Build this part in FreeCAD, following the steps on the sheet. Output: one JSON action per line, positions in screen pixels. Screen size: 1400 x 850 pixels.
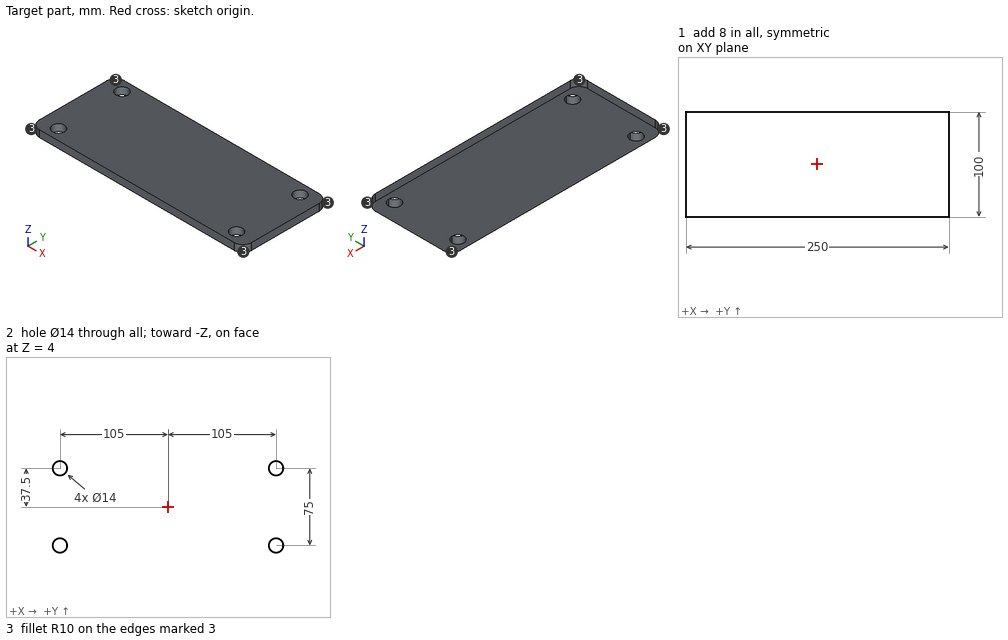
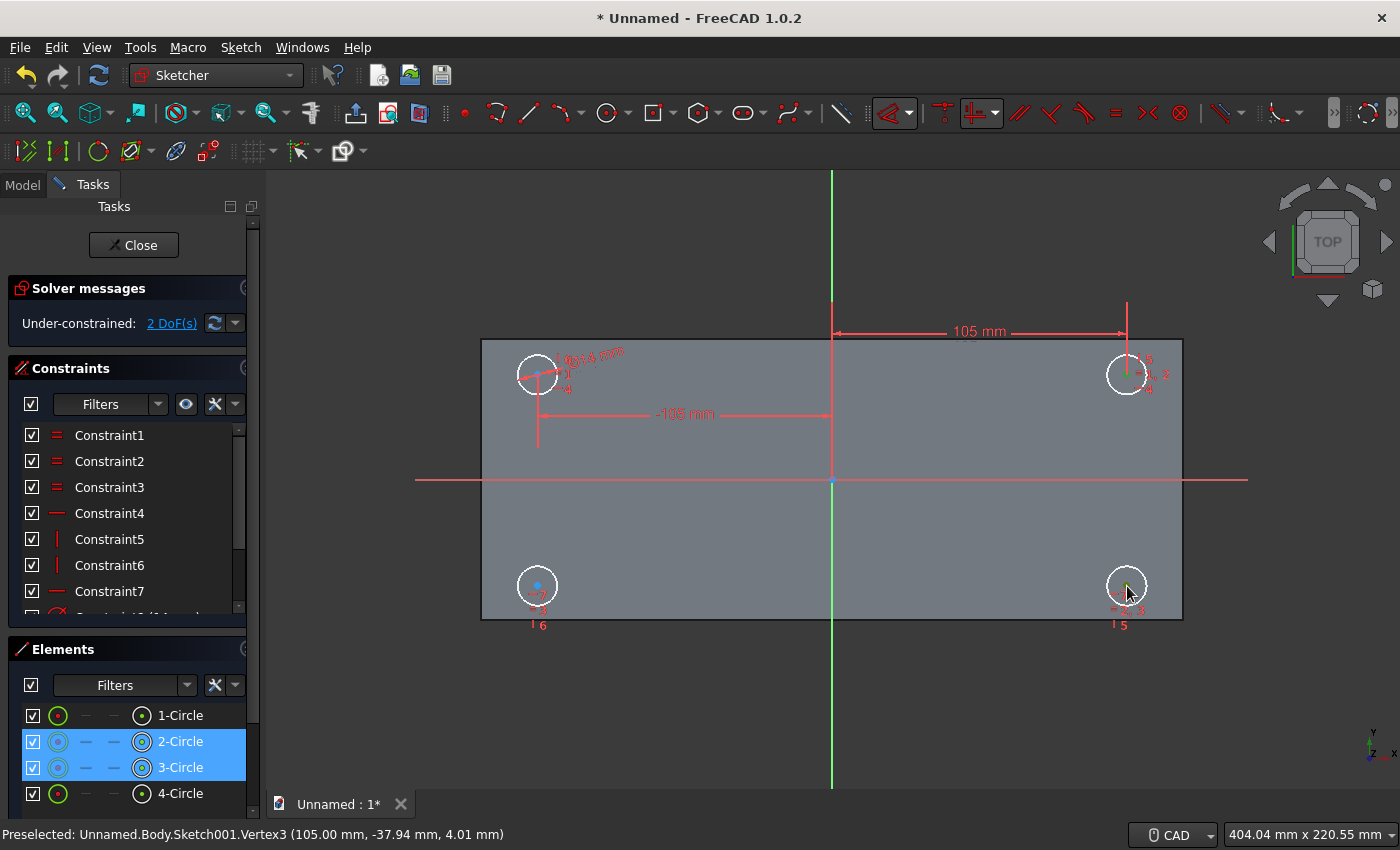
{"action": "left_click", "coordinate": [912, 114]}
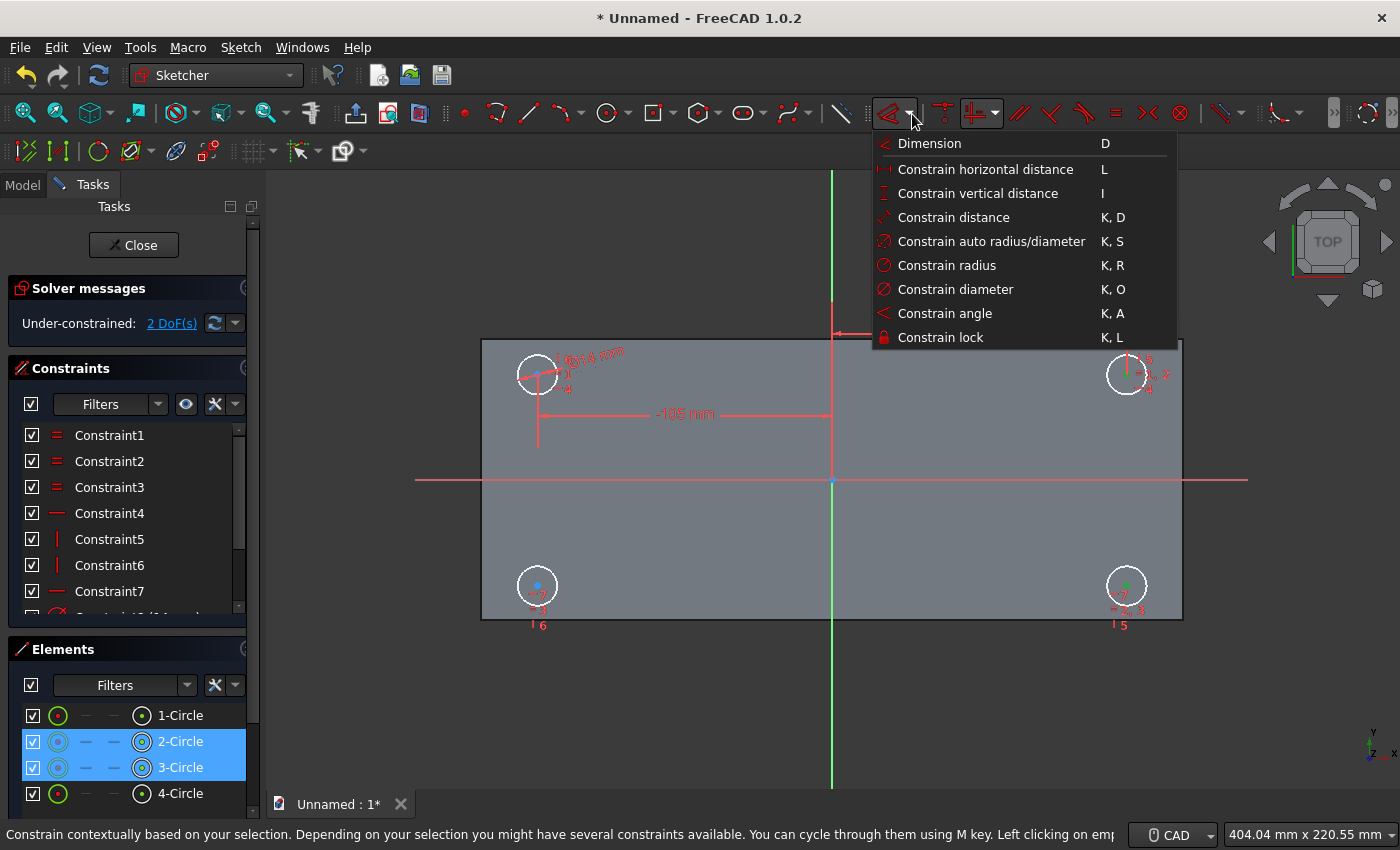
{"action": "left_click", "coordinate": [1025, 193]}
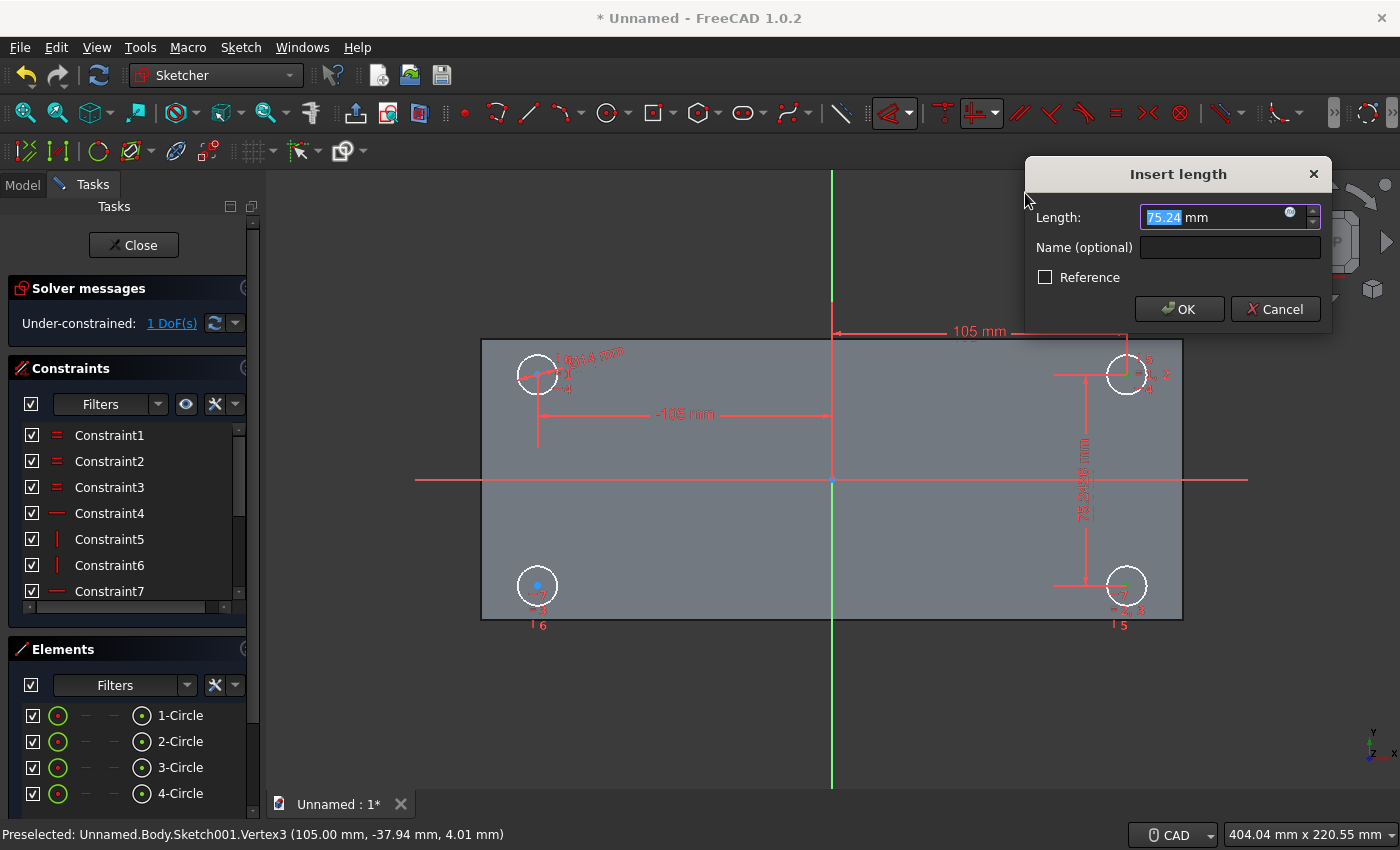
{"action": "type", "text": "75"}
{"action": "key", "text": "Return"}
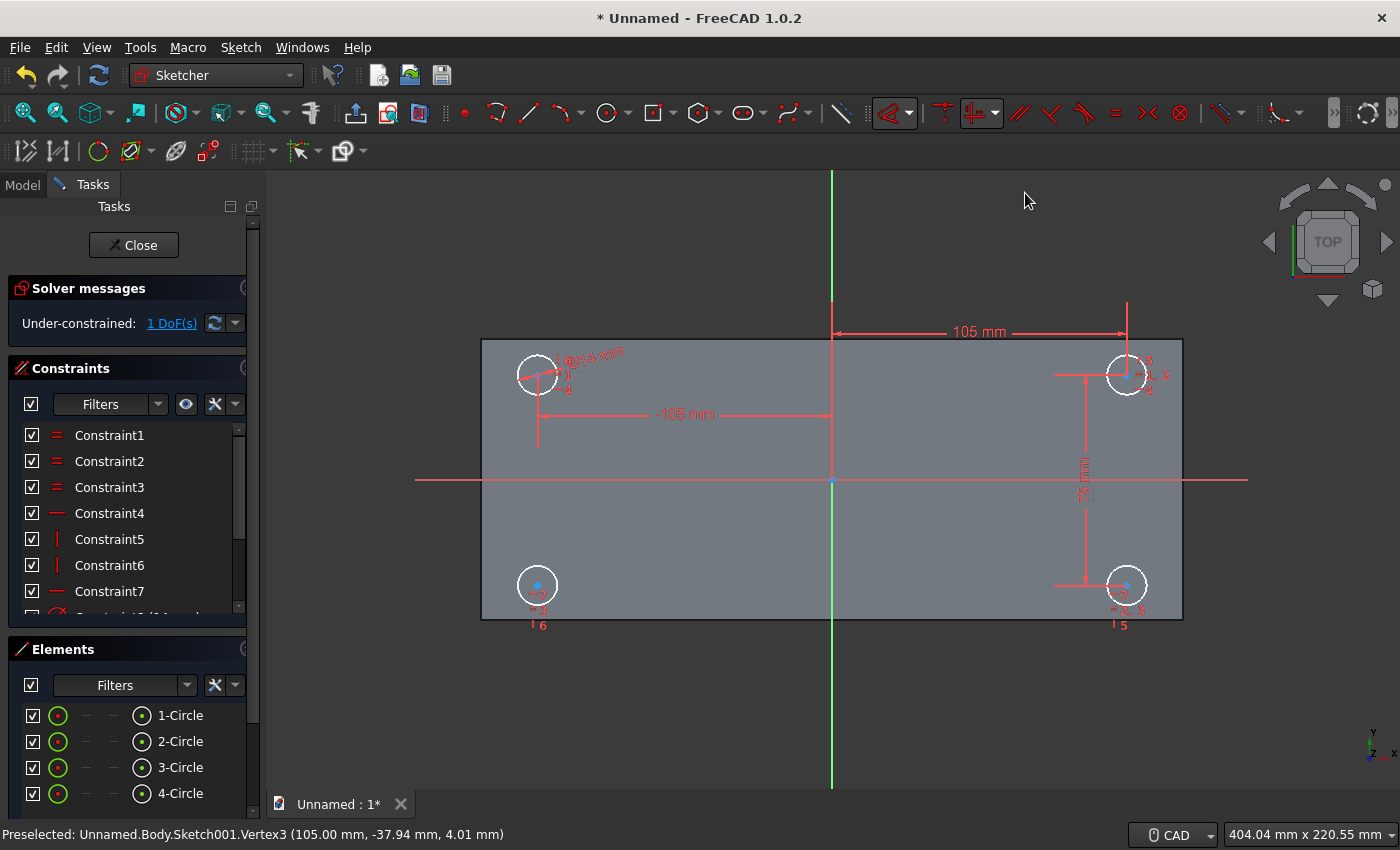
{"action": "left_click", "coordinate": [538, 375]}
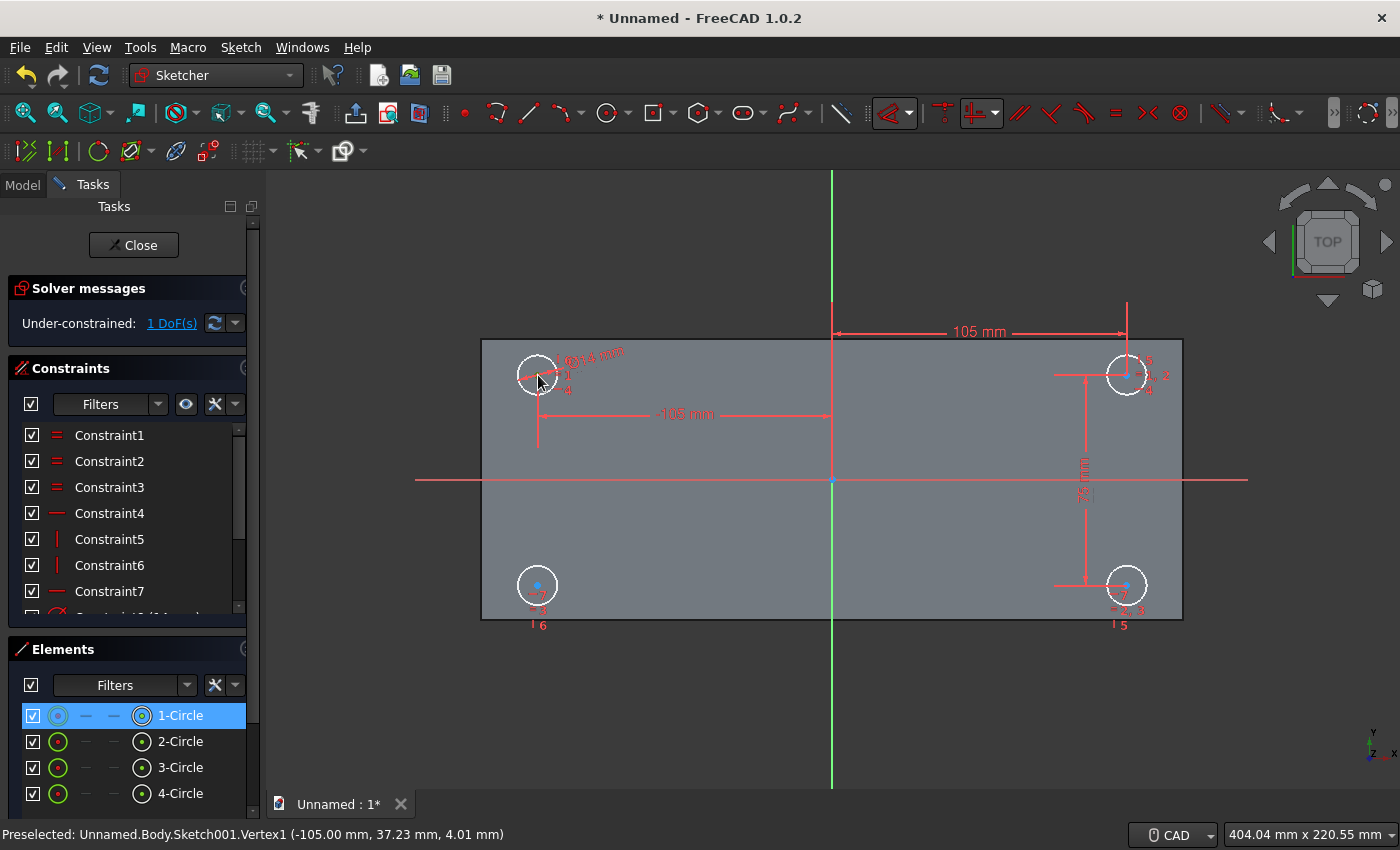
{"action": "key", "text": "i"}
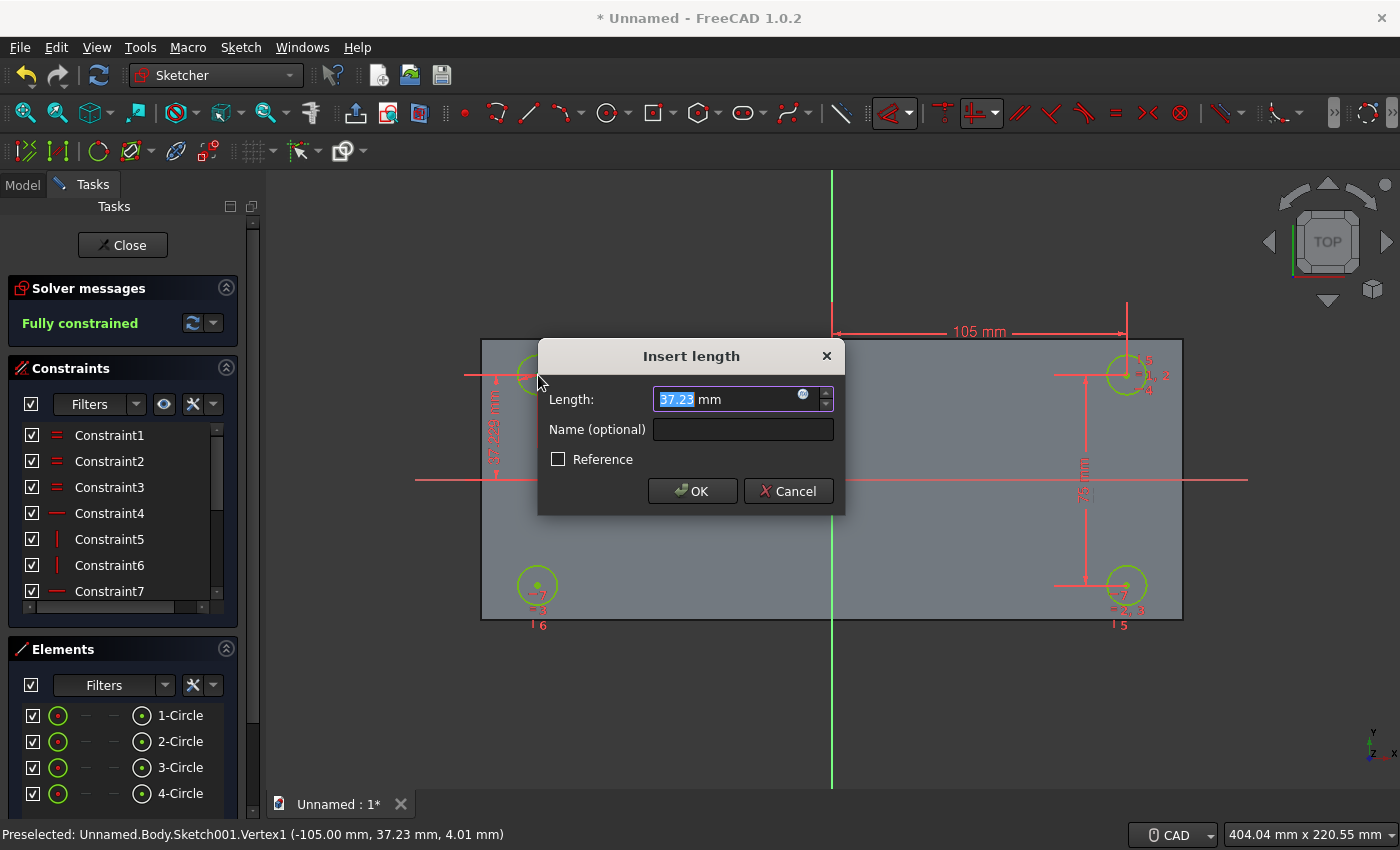
{"action": "type", "text": "37.5"}
{"action": "key", "text": "Return"}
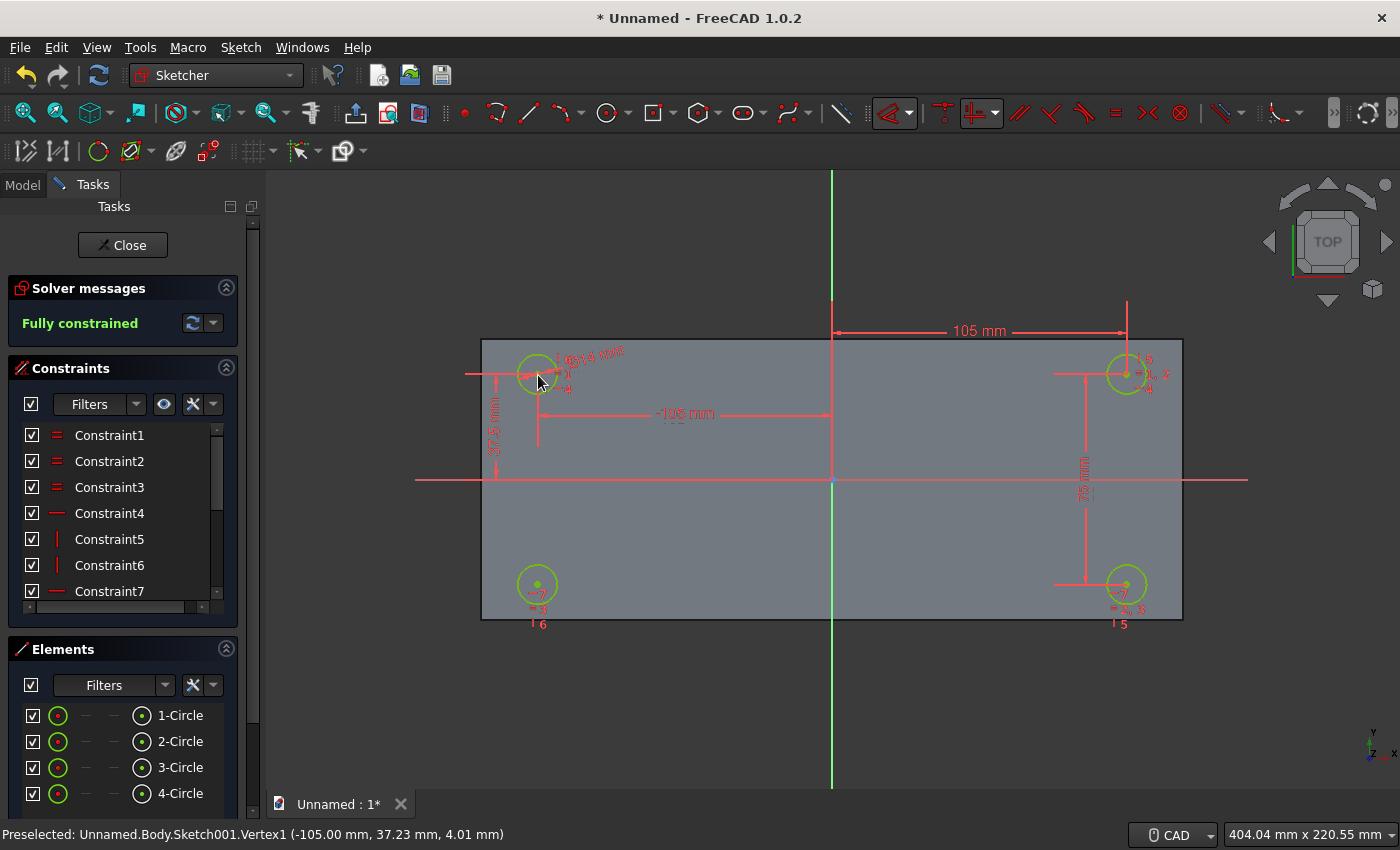
{"action": "left_click", "coordinate": [123, 245]}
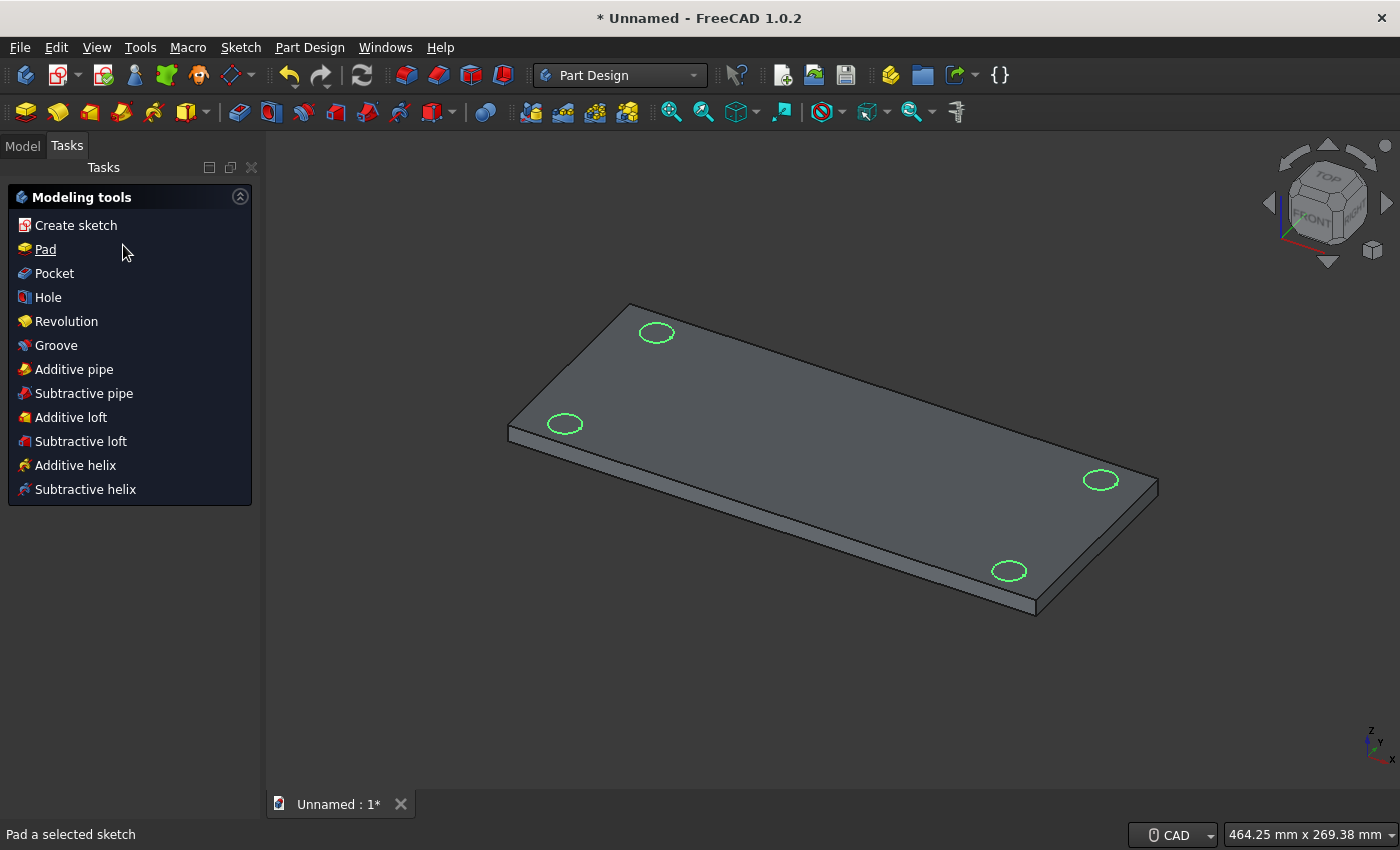
{"action": "left_click", "coordinate": [272, 112]}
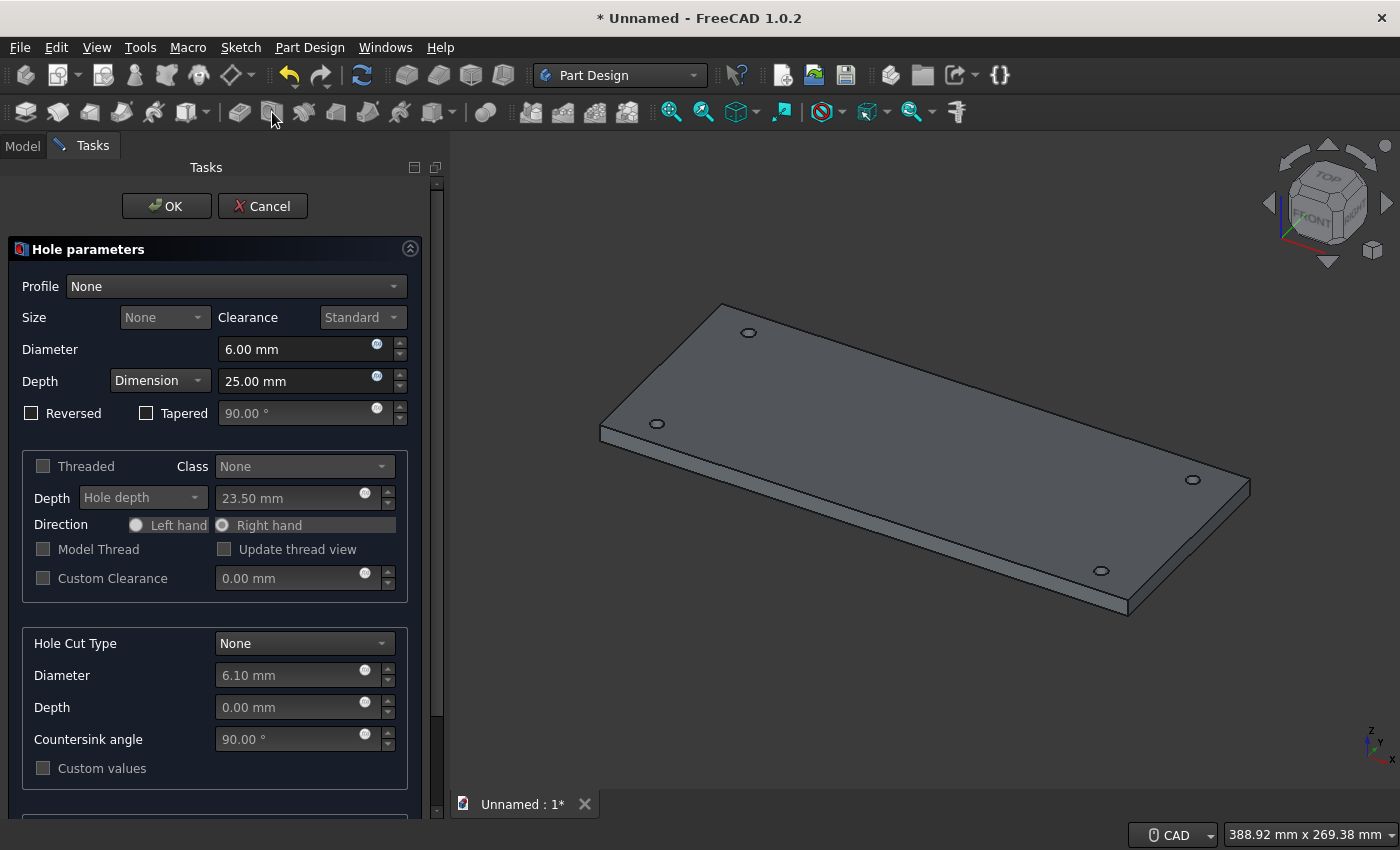
{"action": "triple_click", "coordinate": [305, 349]}